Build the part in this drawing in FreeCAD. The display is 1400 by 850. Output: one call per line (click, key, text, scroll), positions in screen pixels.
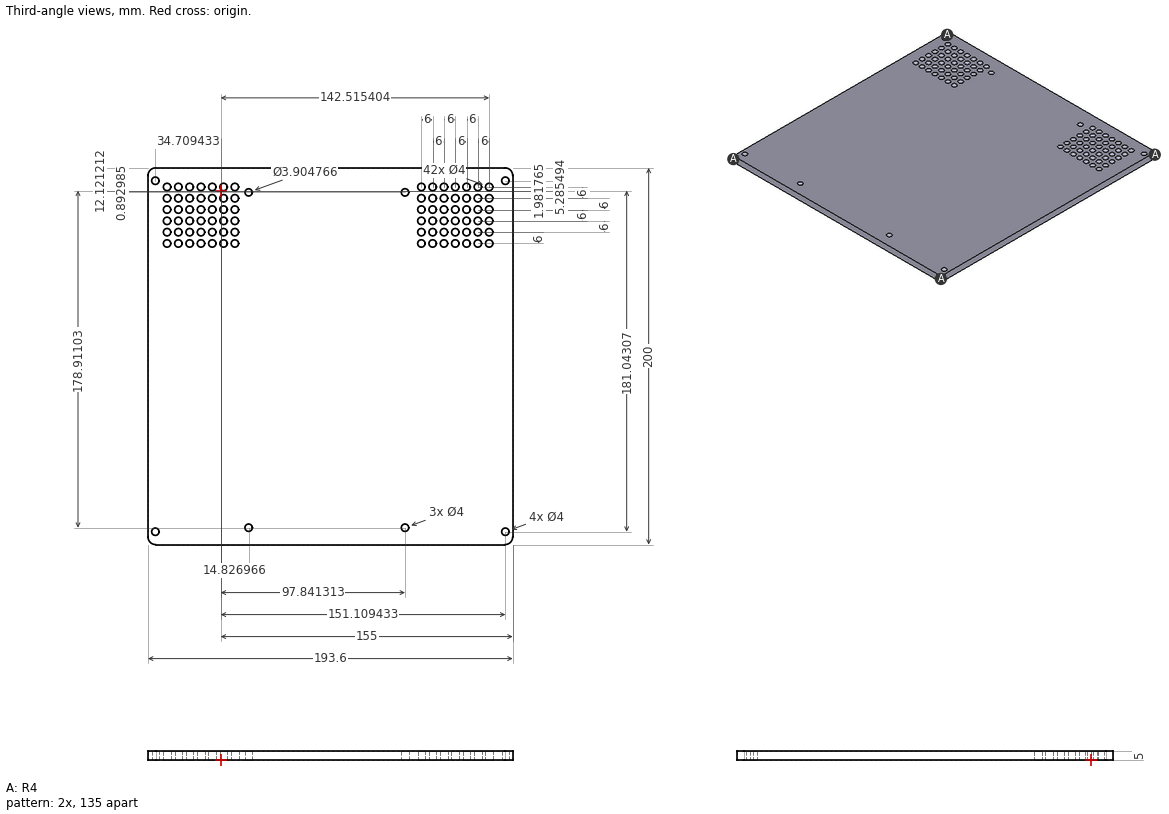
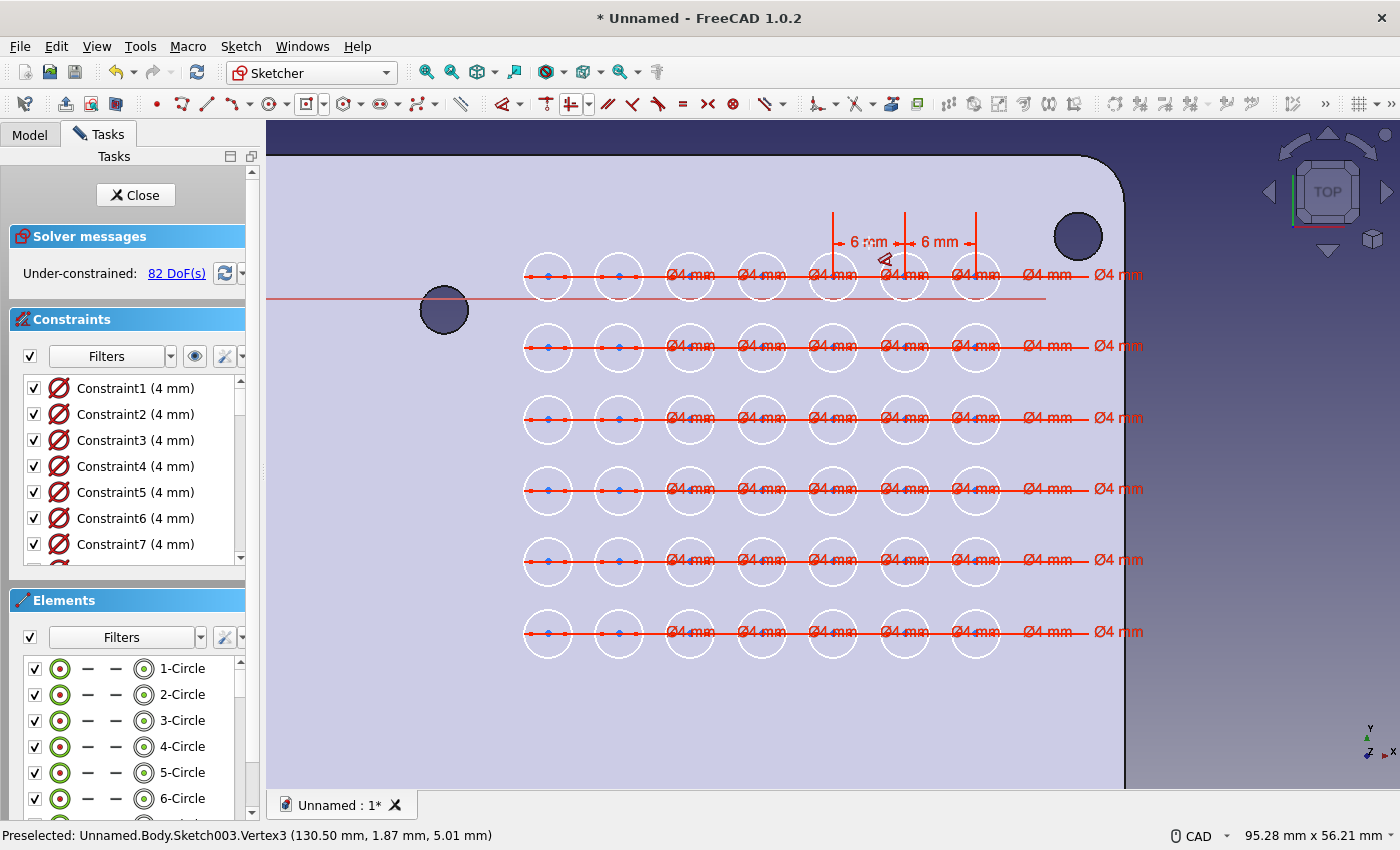
click(833, 277)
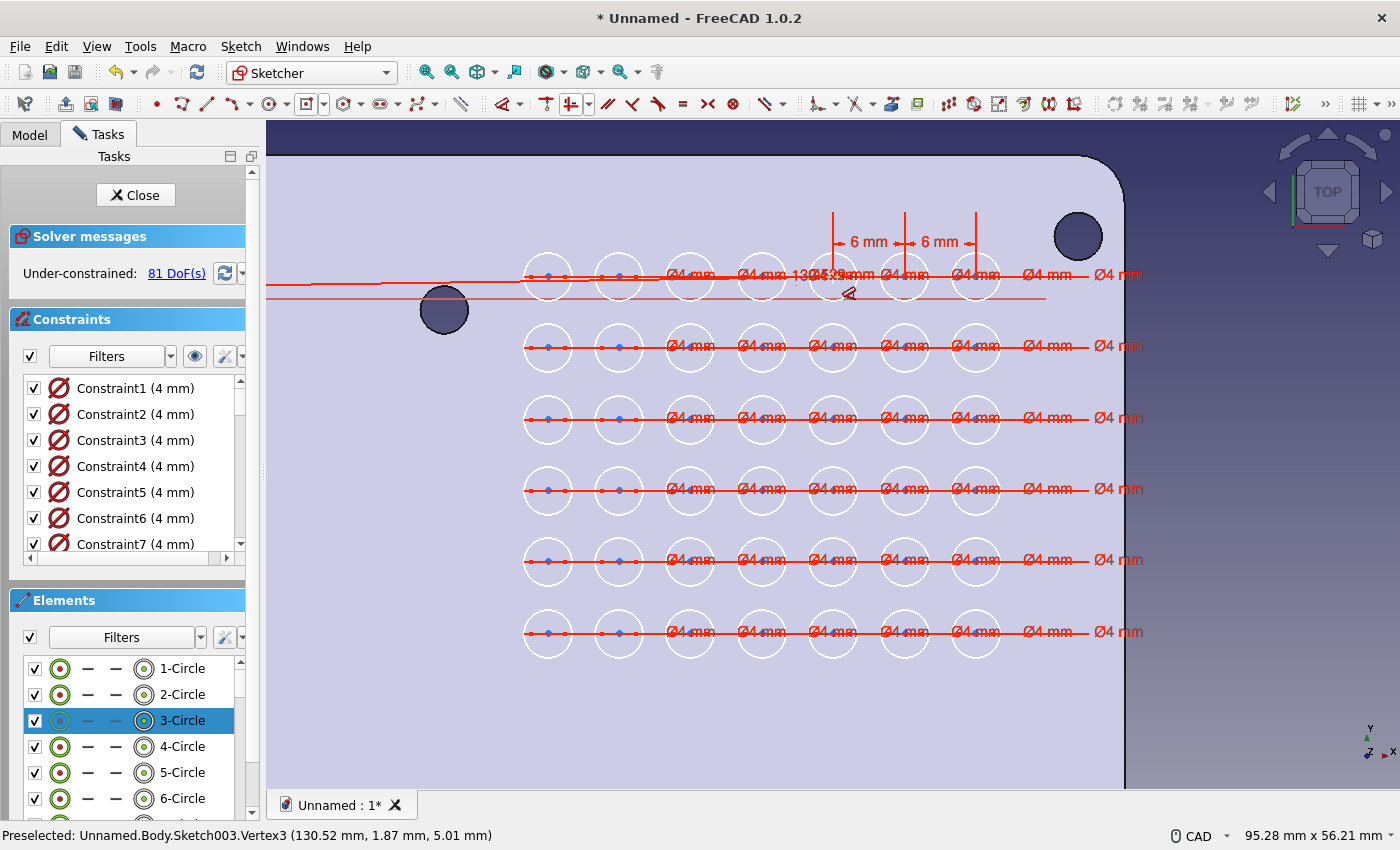
click(762, 277)
click(798, 243)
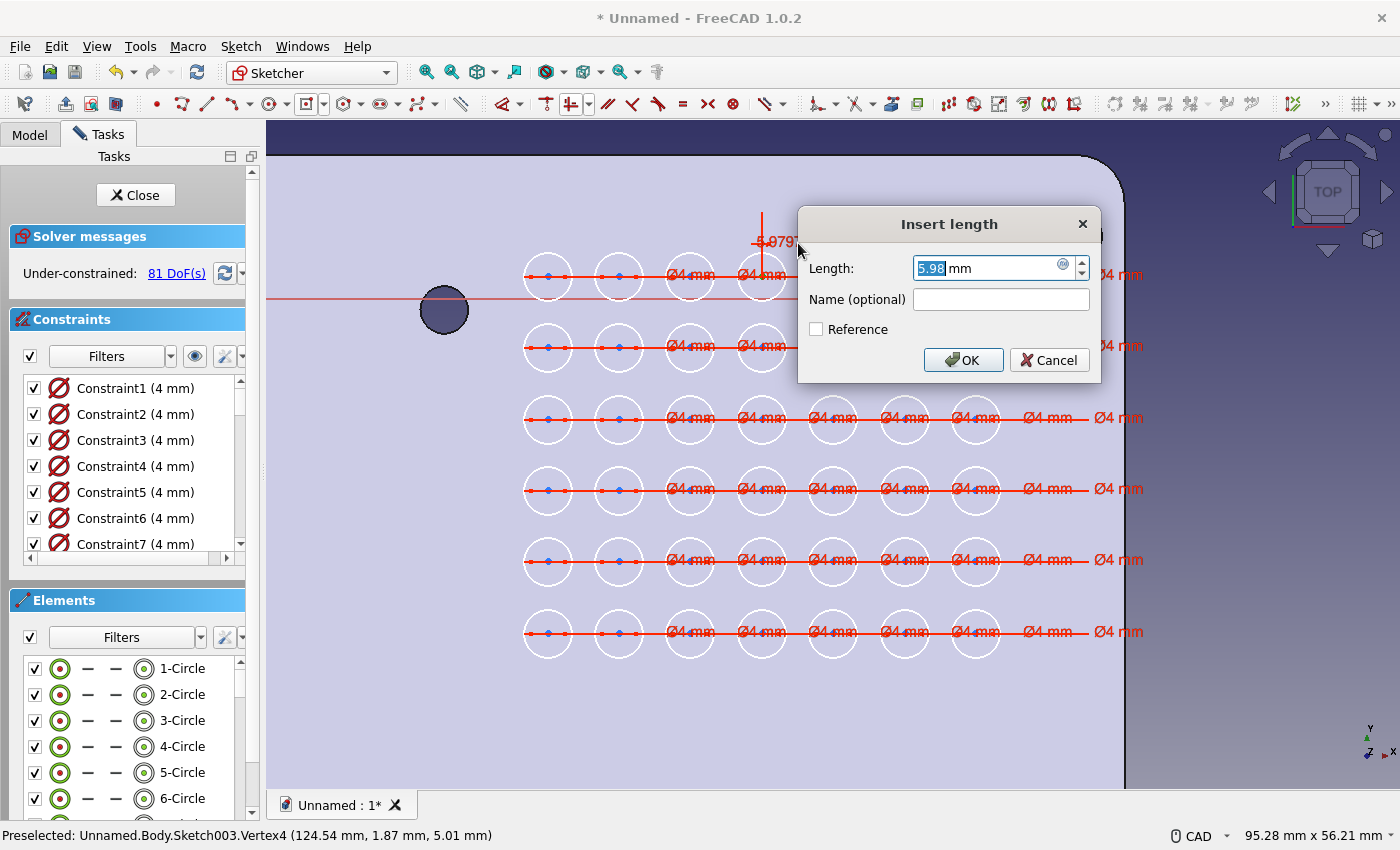
text(6)
key(Return)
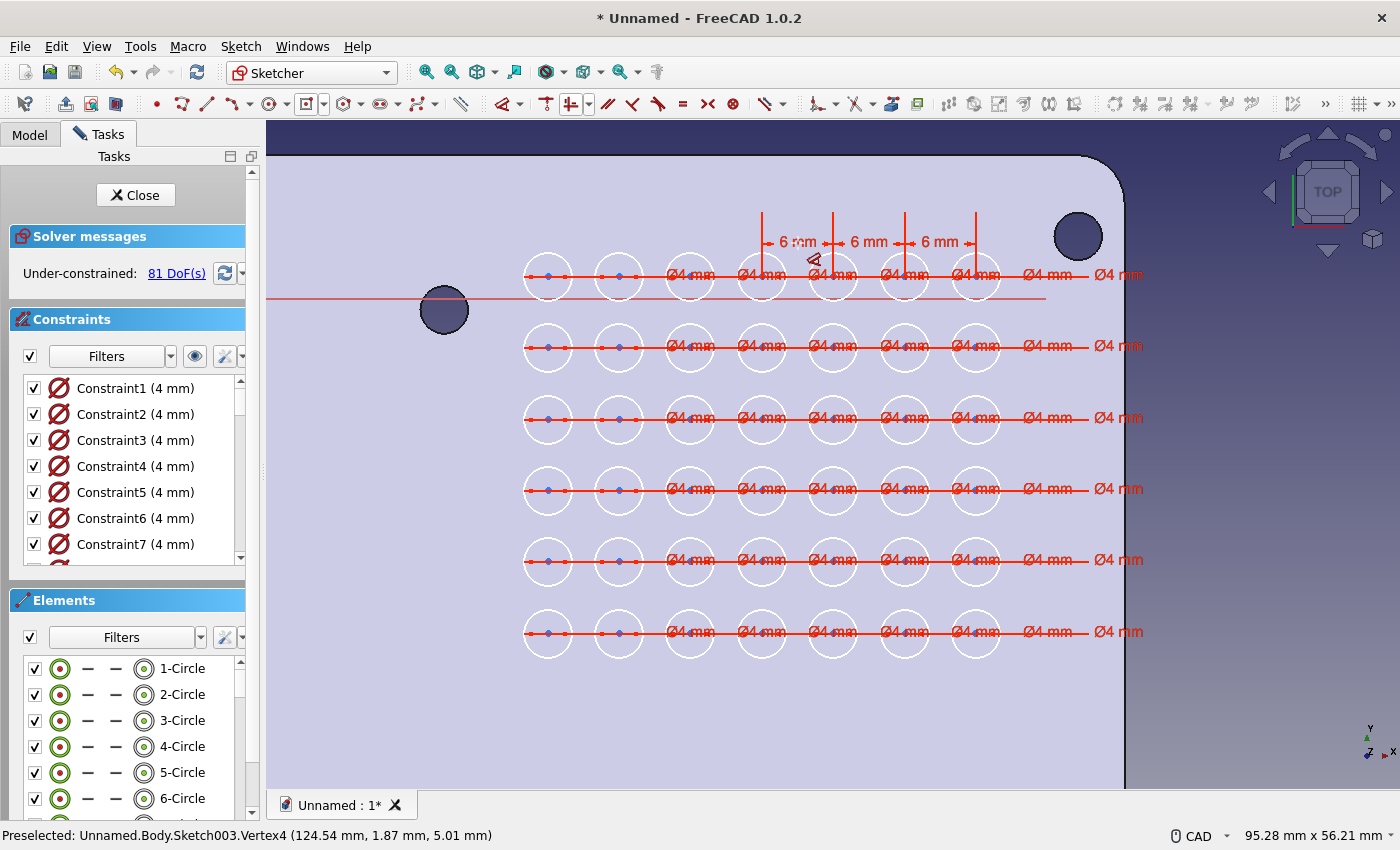
click(762, 277)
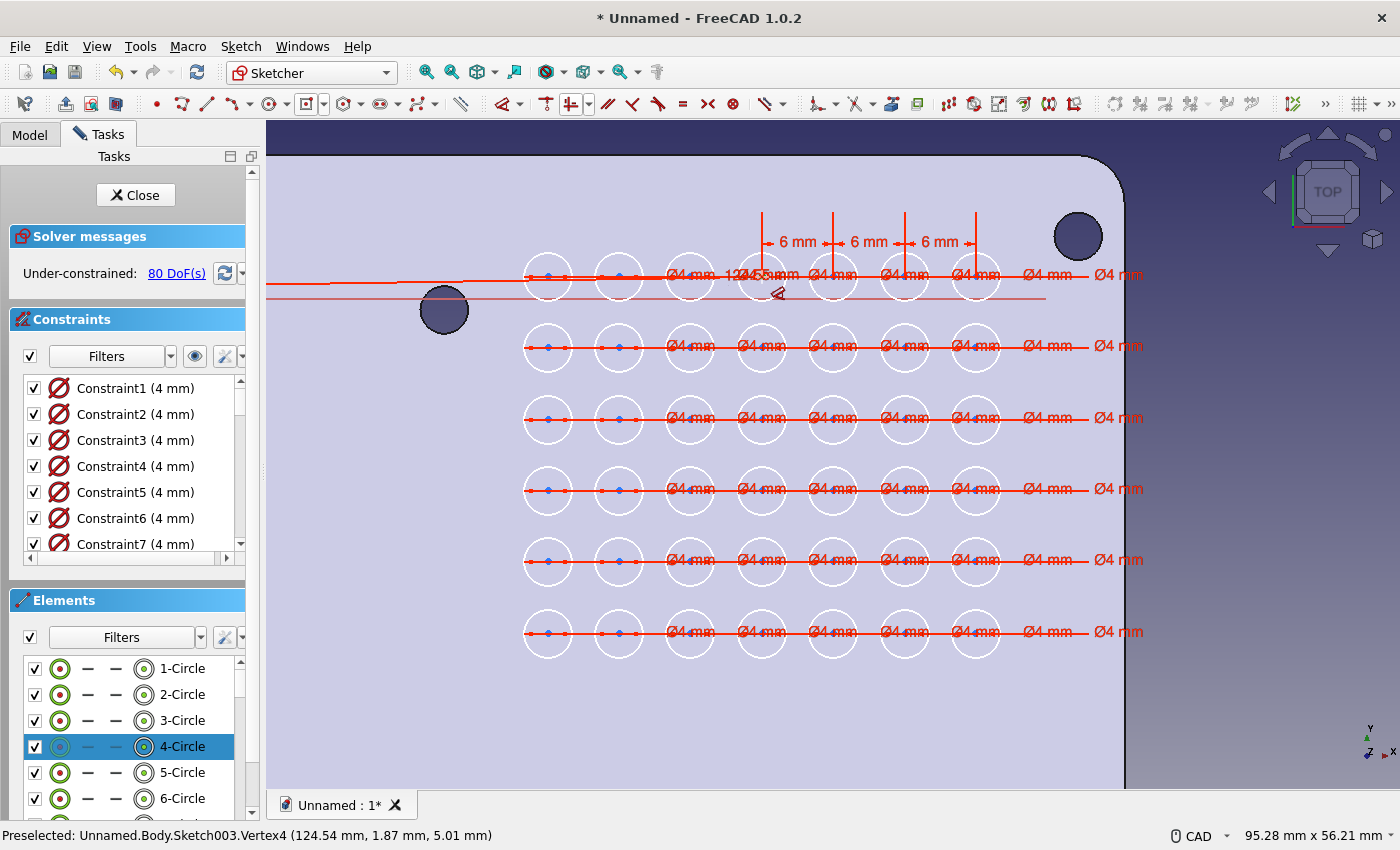
click(690, 277)
click(726, 243)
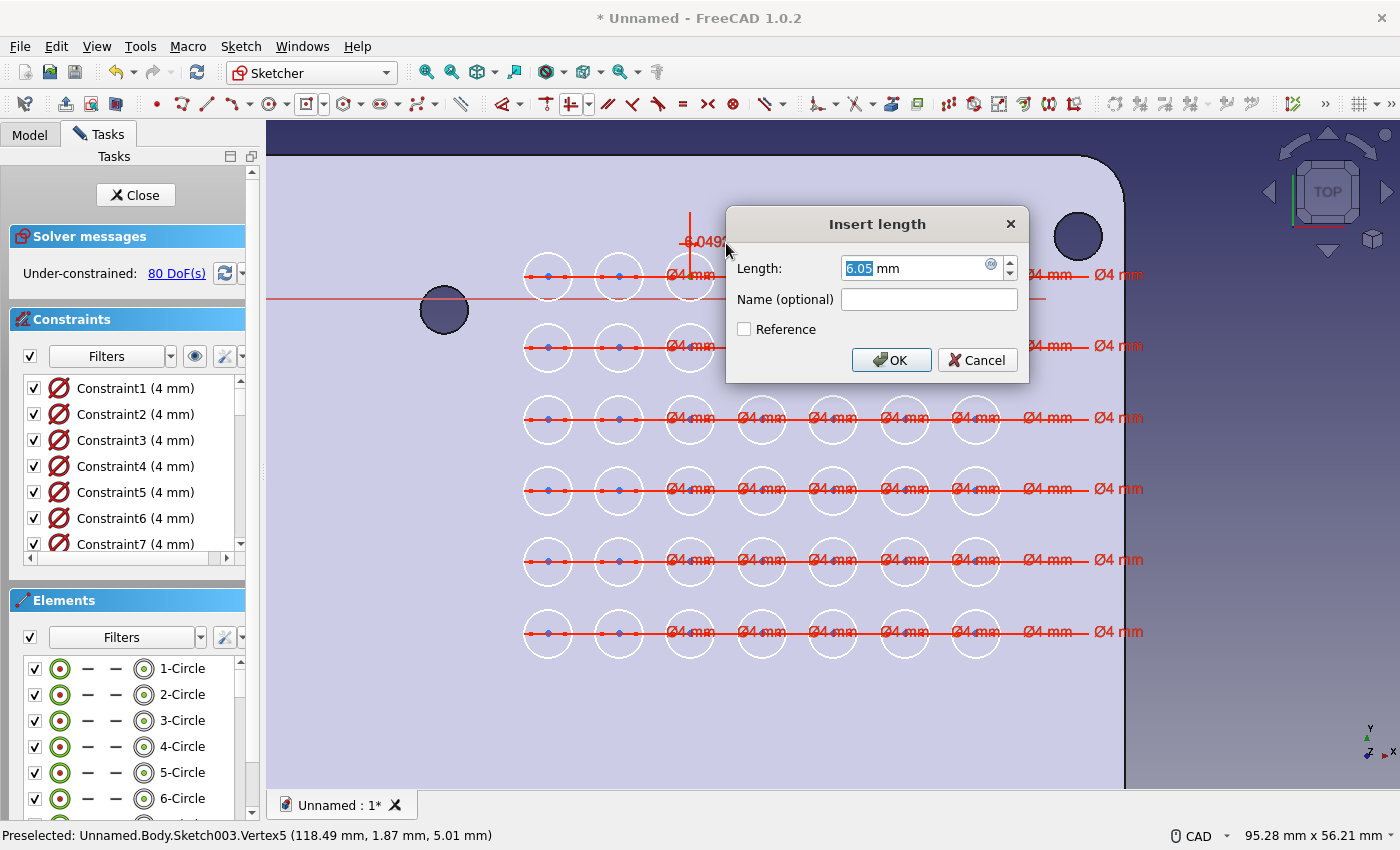
text(6)
key(Return)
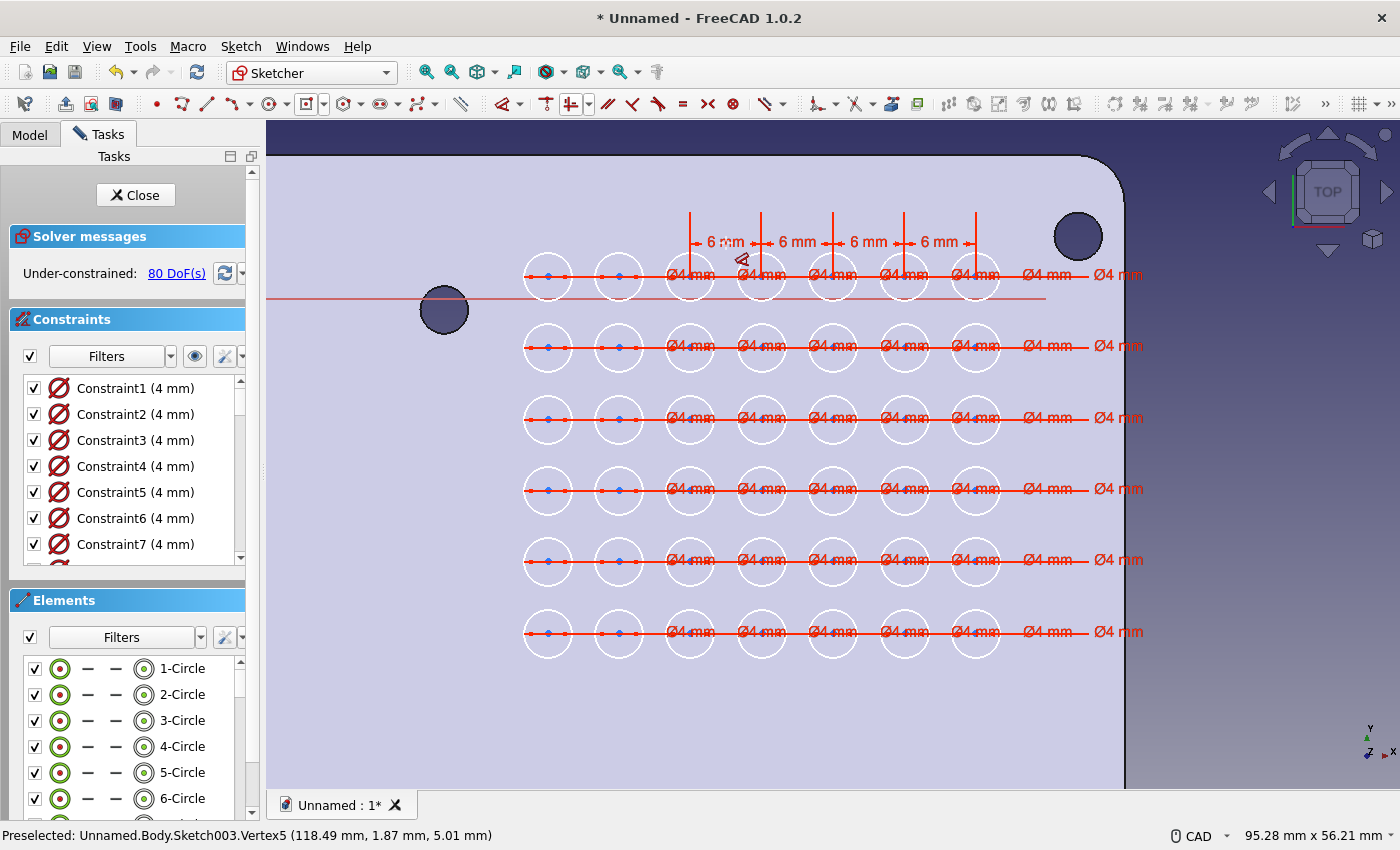
click(690, 277)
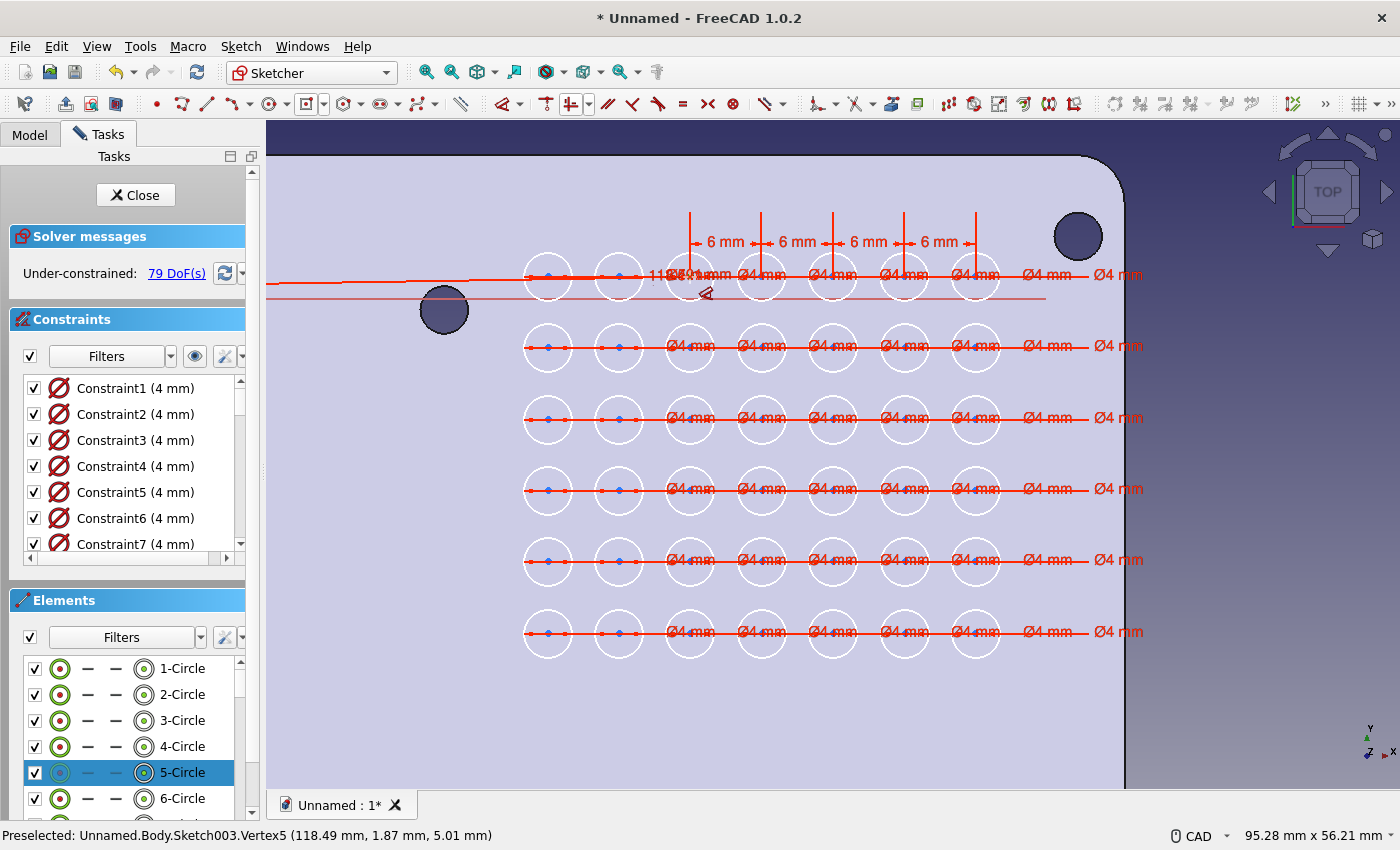
click(619, 277)
click(654, 243)